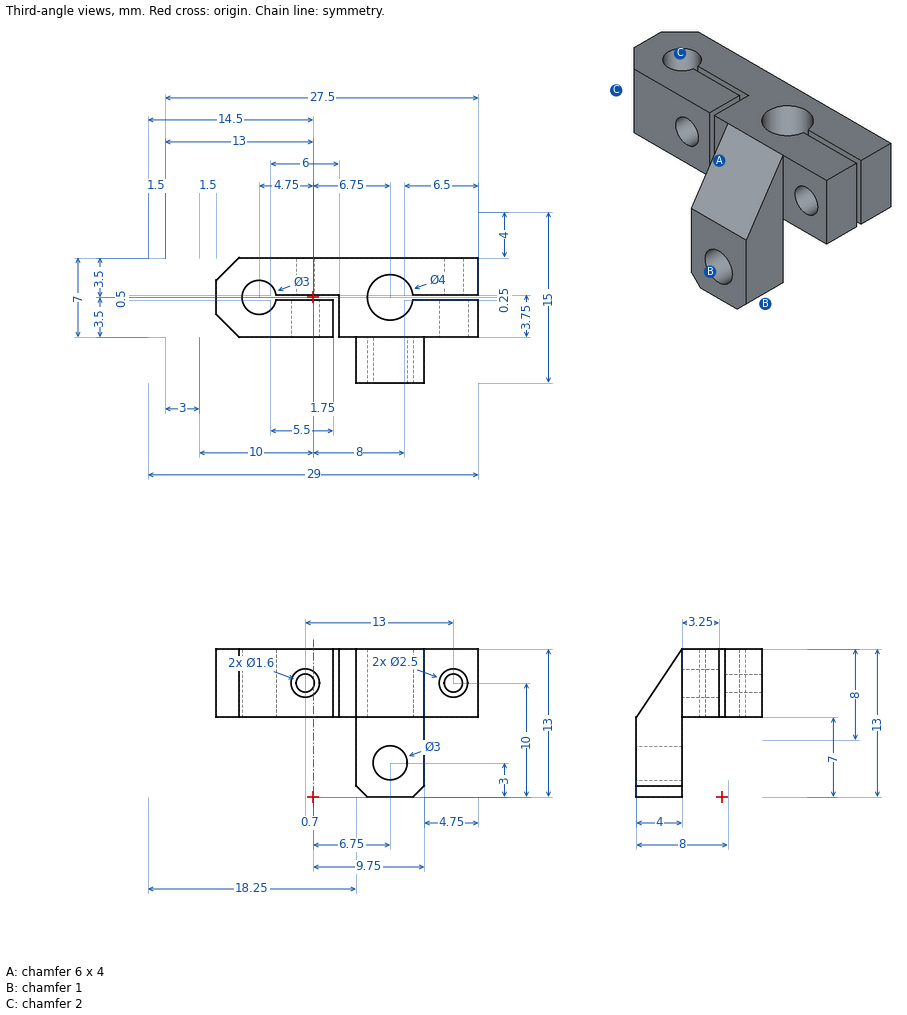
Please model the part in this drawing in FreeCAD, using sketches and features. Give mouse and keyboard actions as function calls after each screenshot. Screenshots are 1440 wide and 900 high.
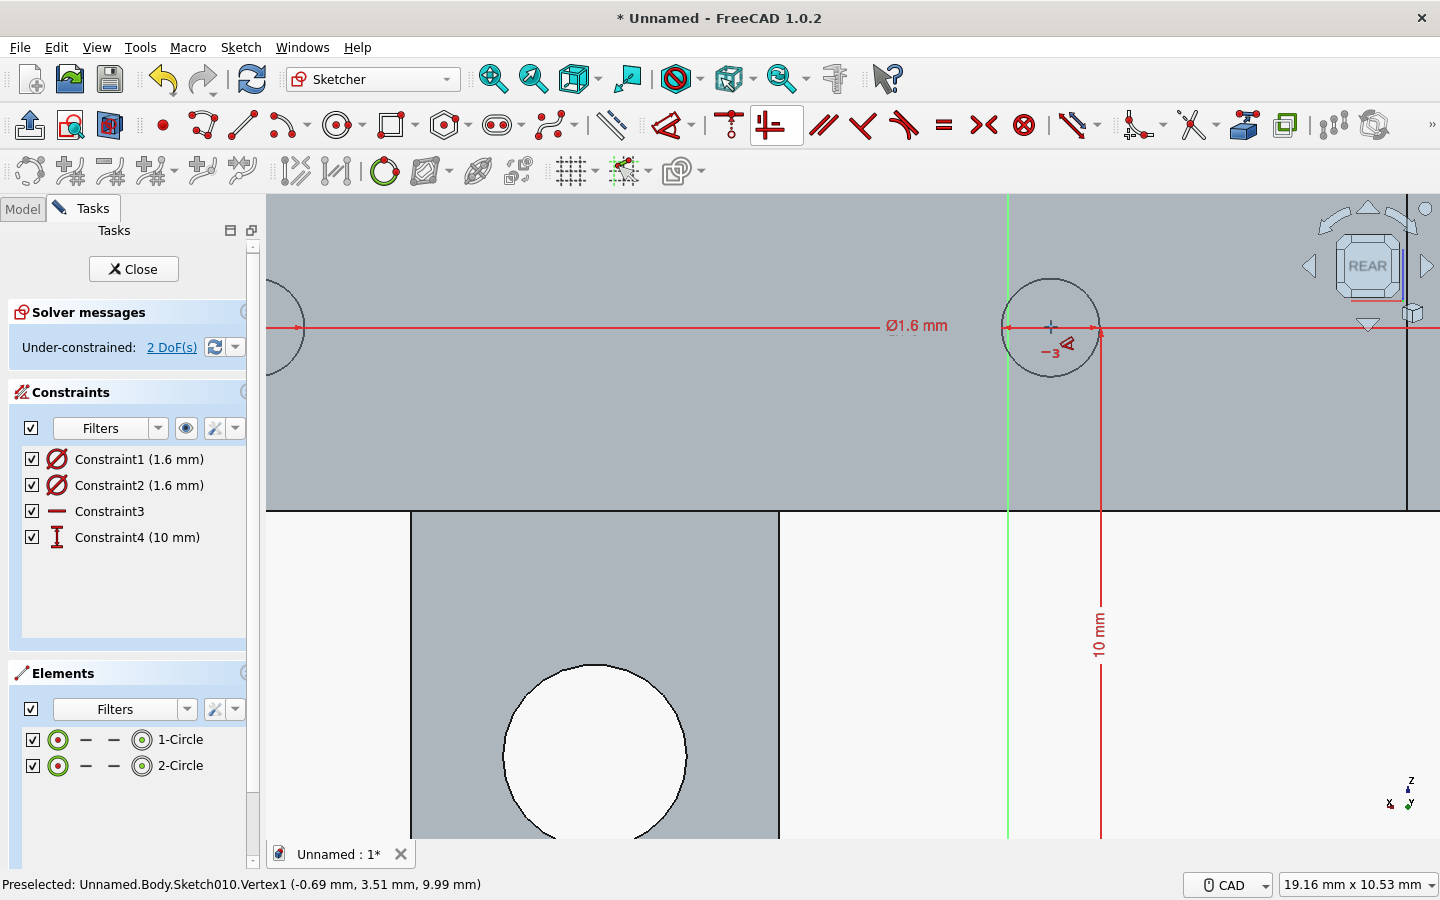
click(1051, 328)
click(1039, 294)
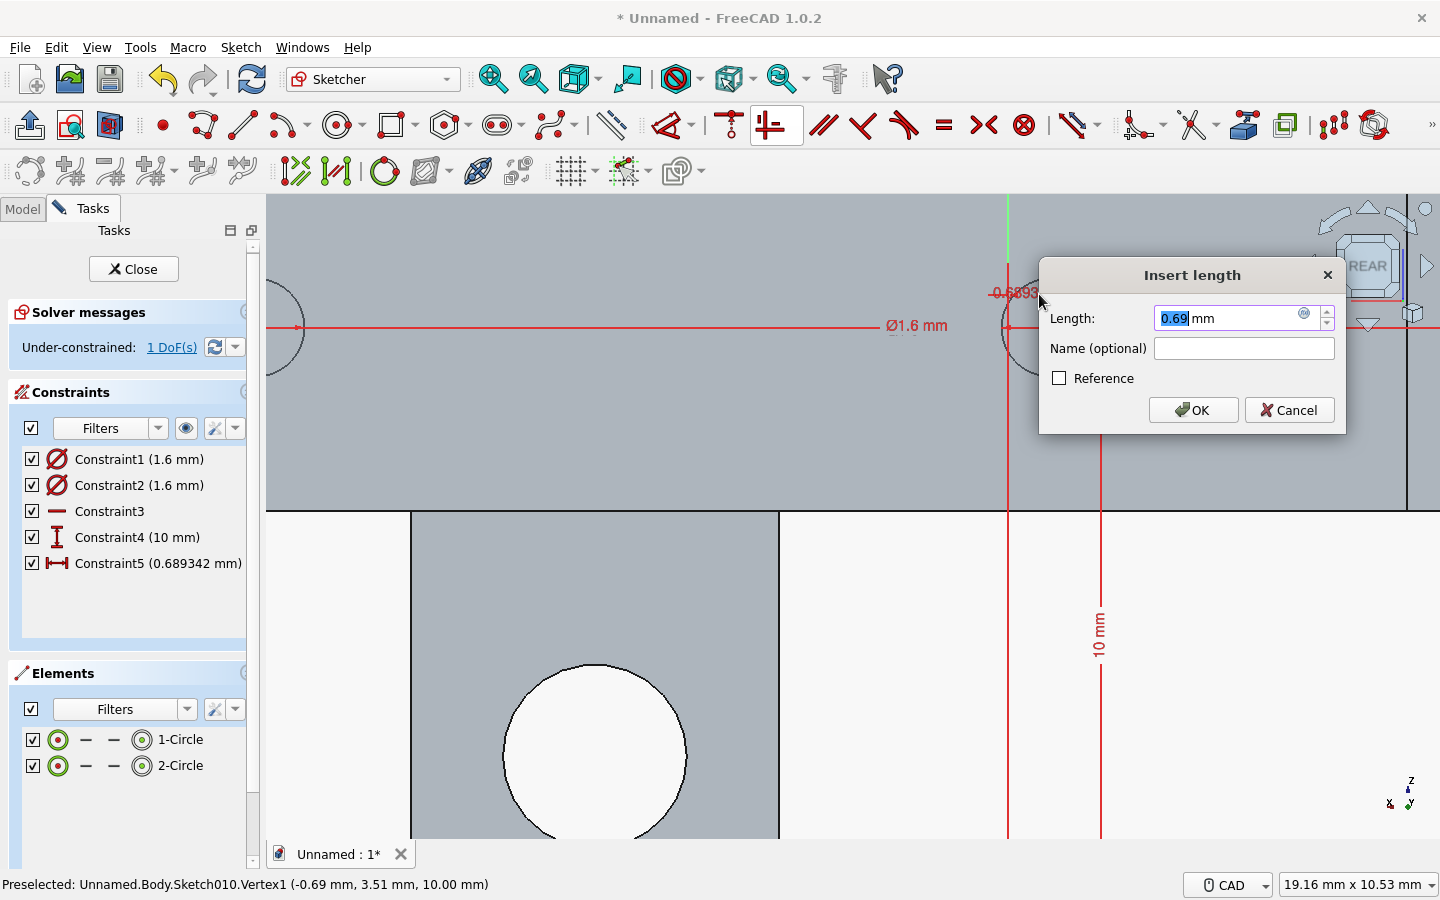
text(0.7)
key(Return)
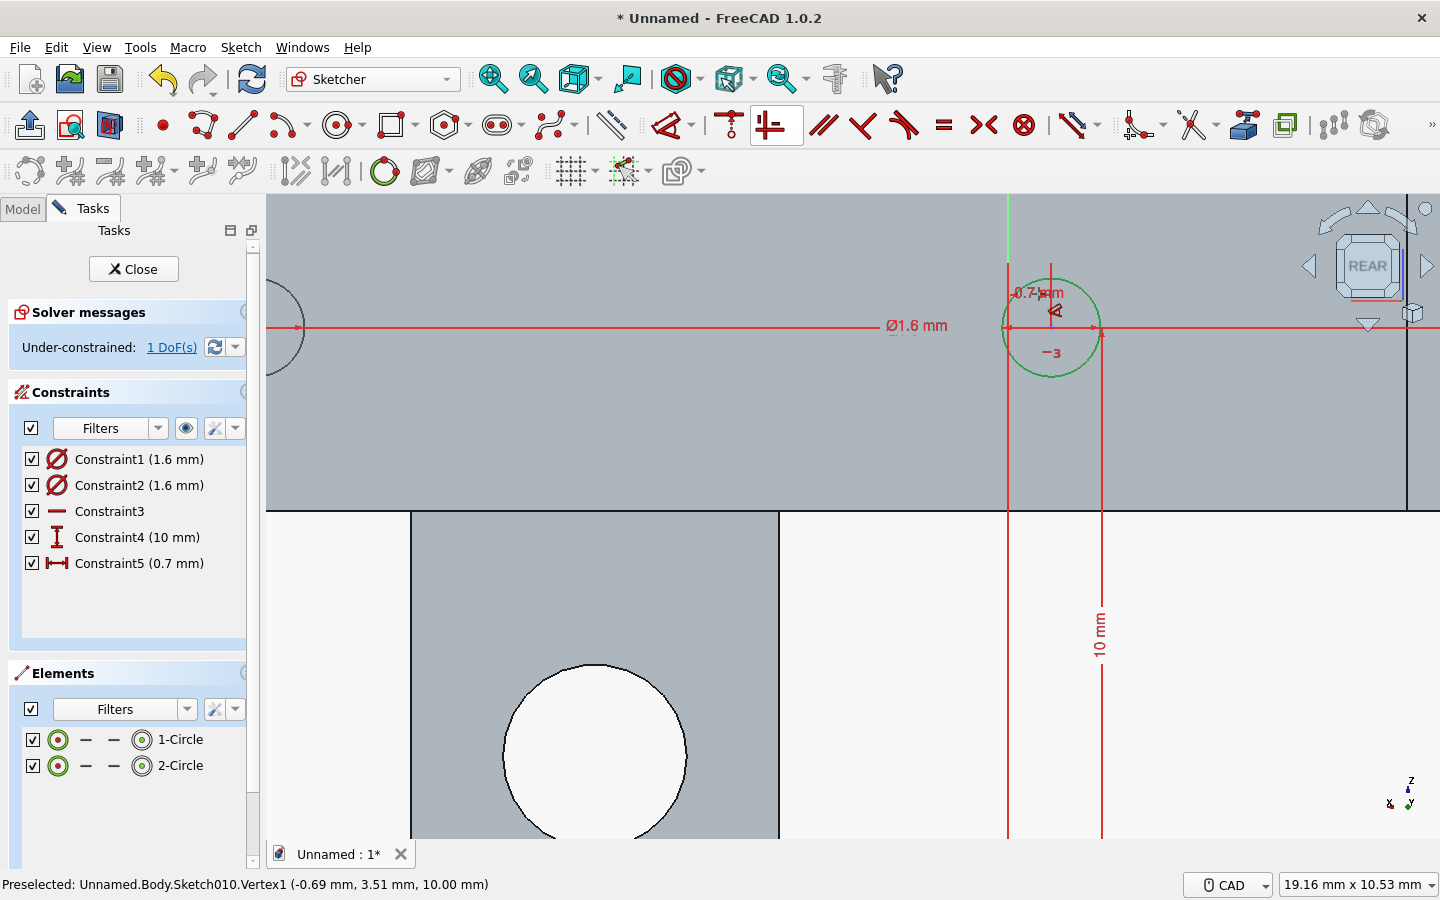
click(1051, 328)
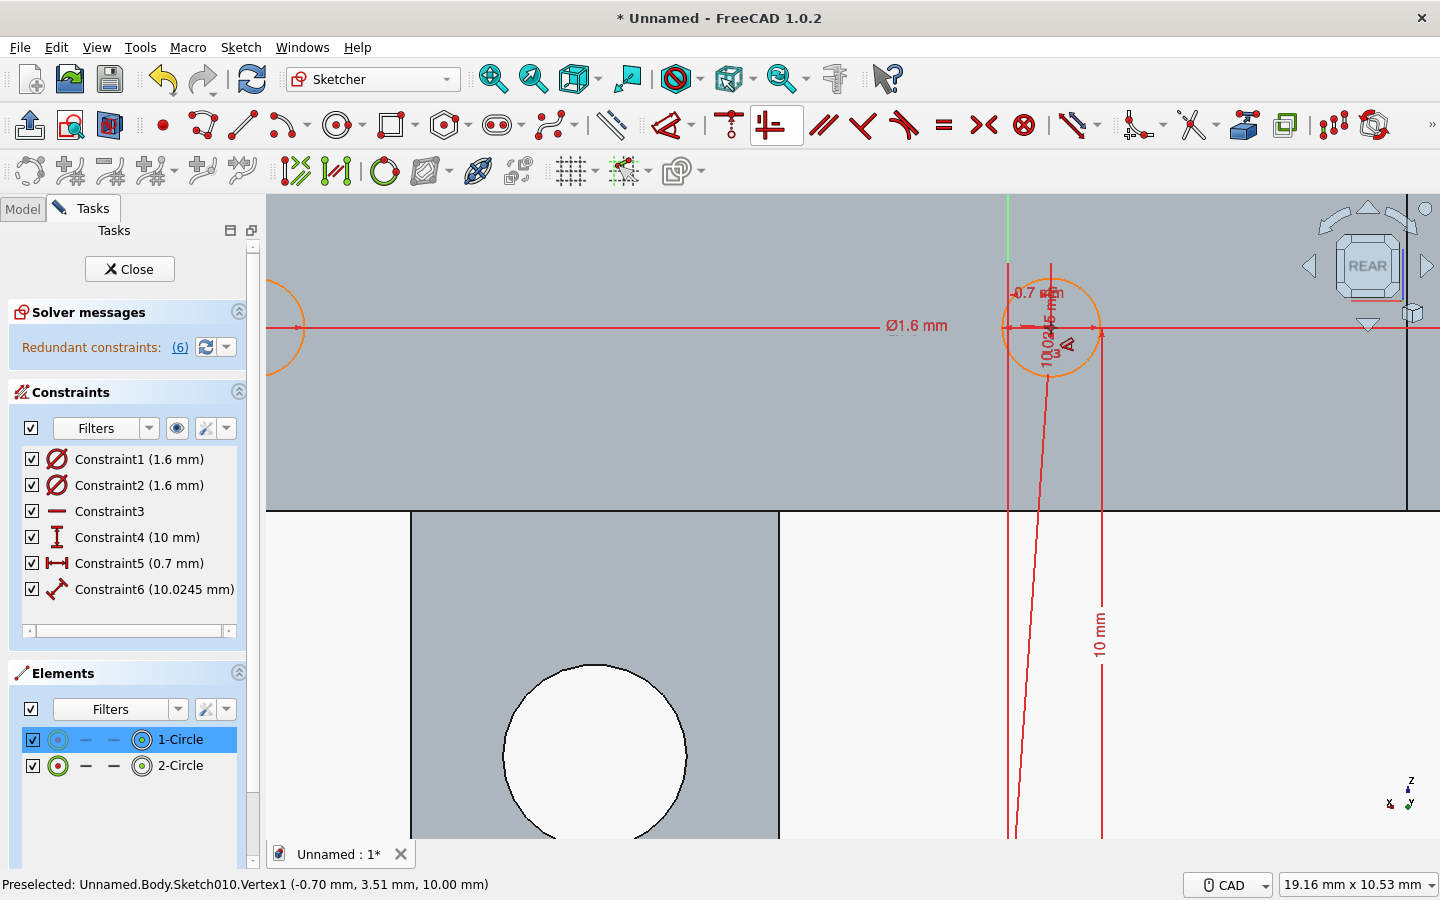
scroll(1052, 328, down, 2)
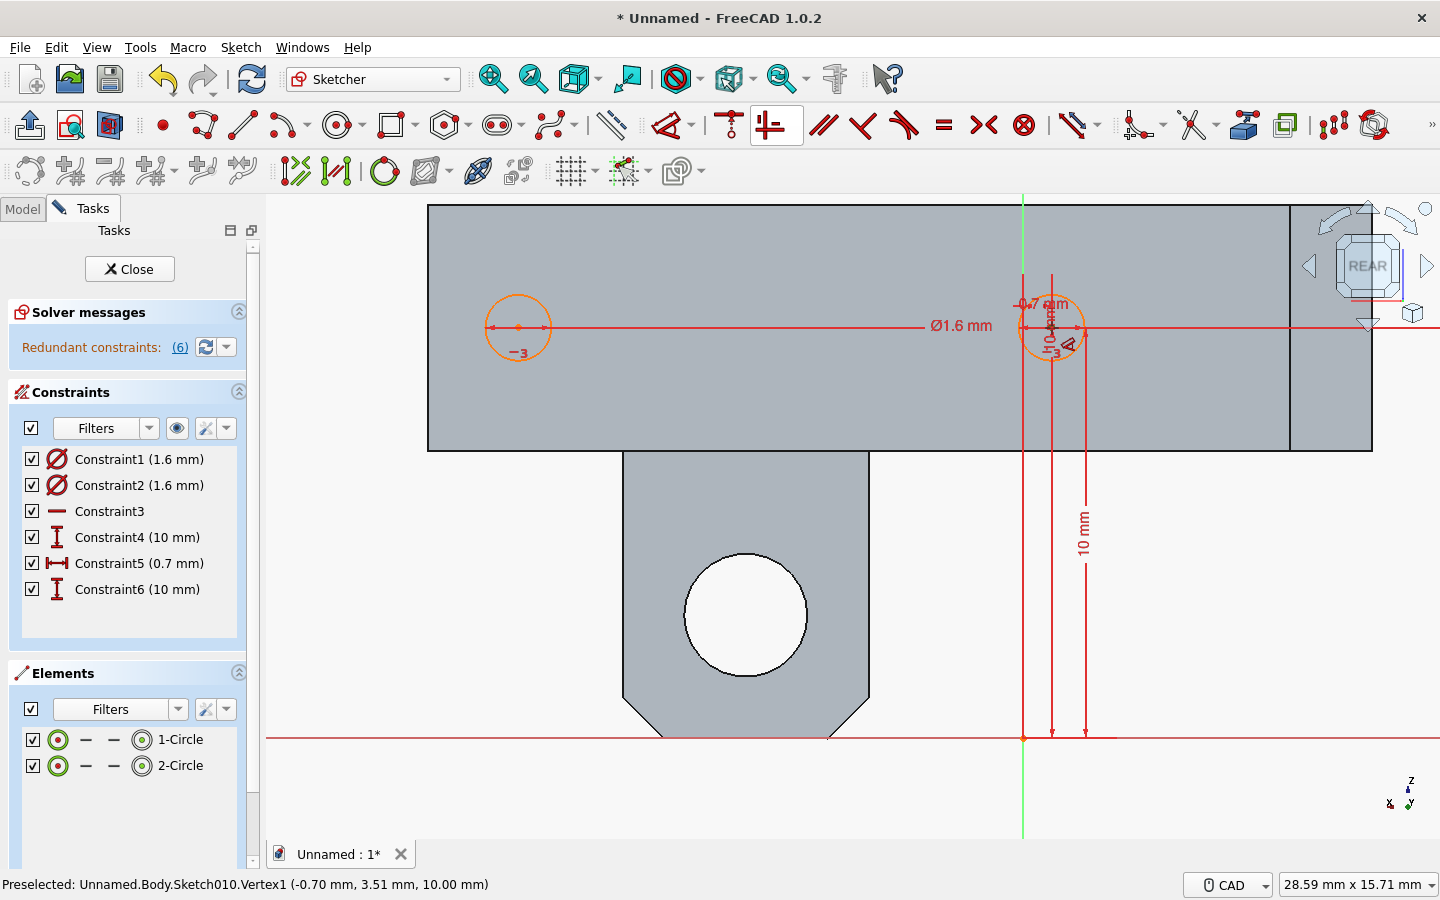
click(518, 328)
click(785, 294)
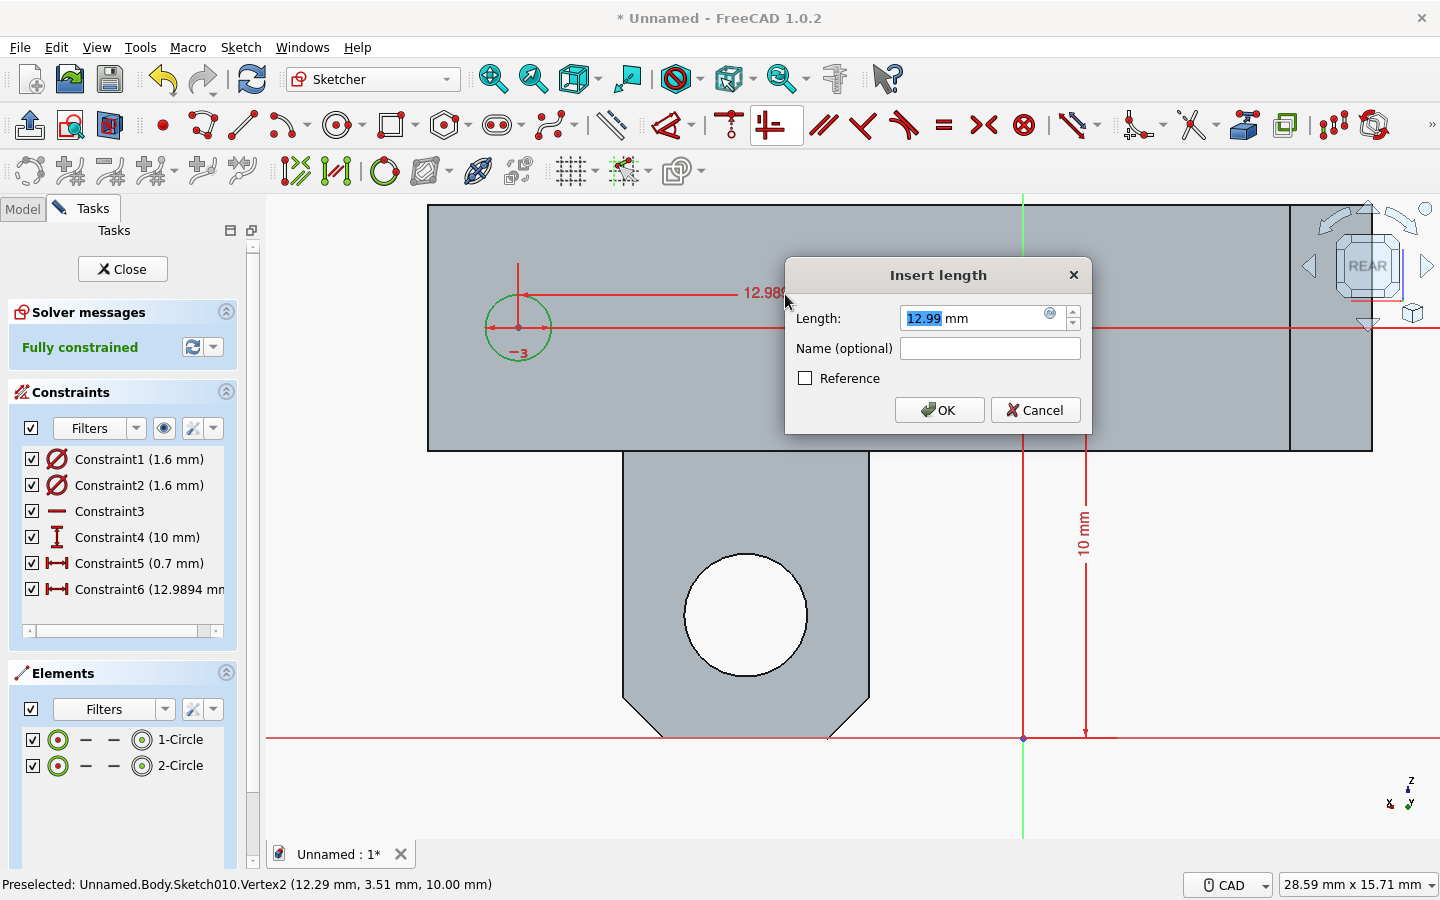
text(13)
key(Return)
key(Escape)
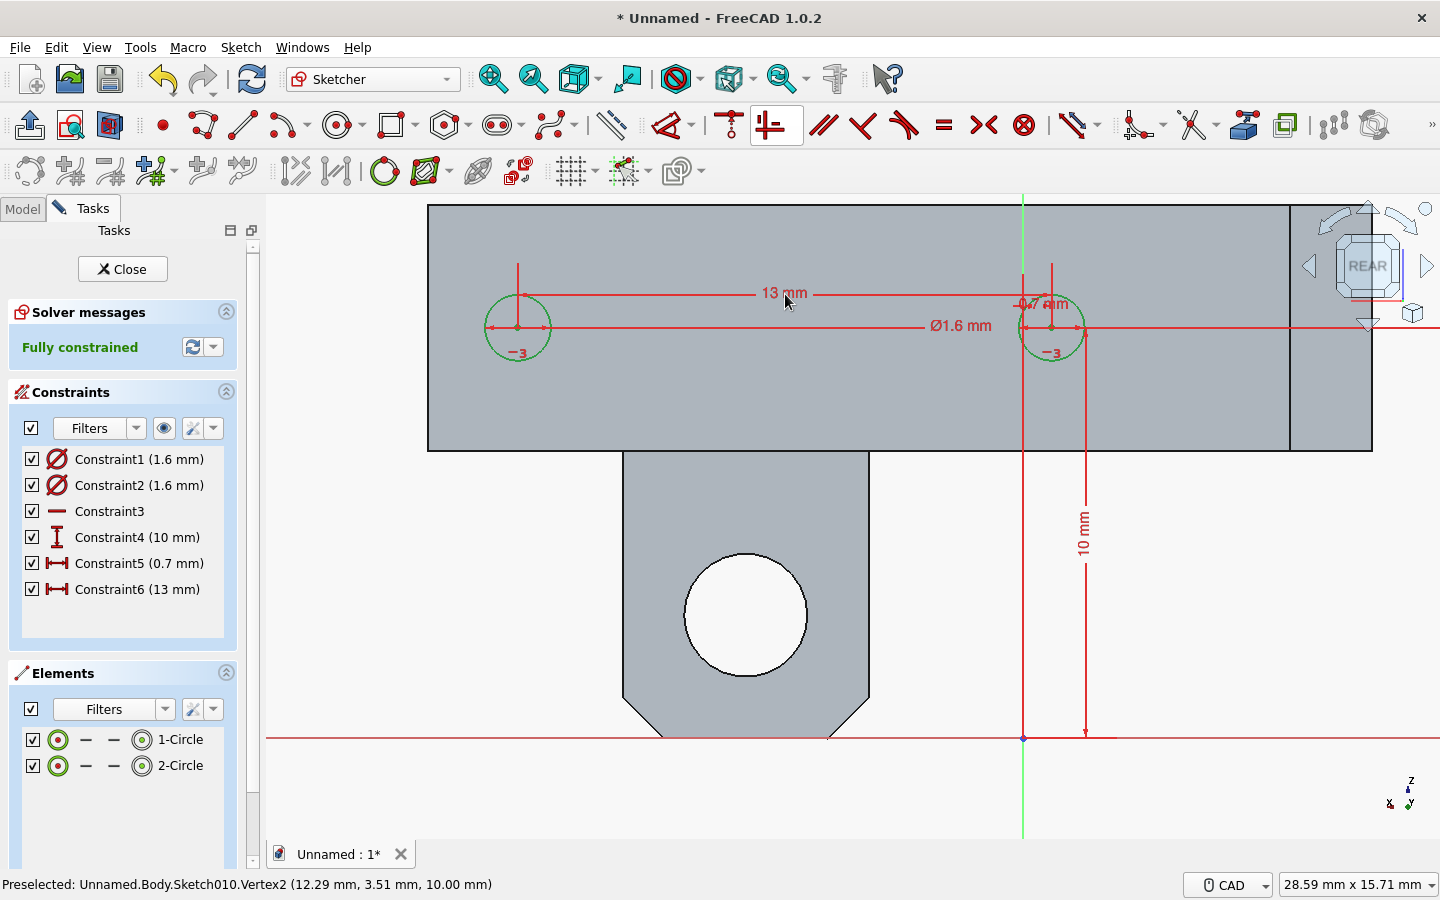
click(123, 269)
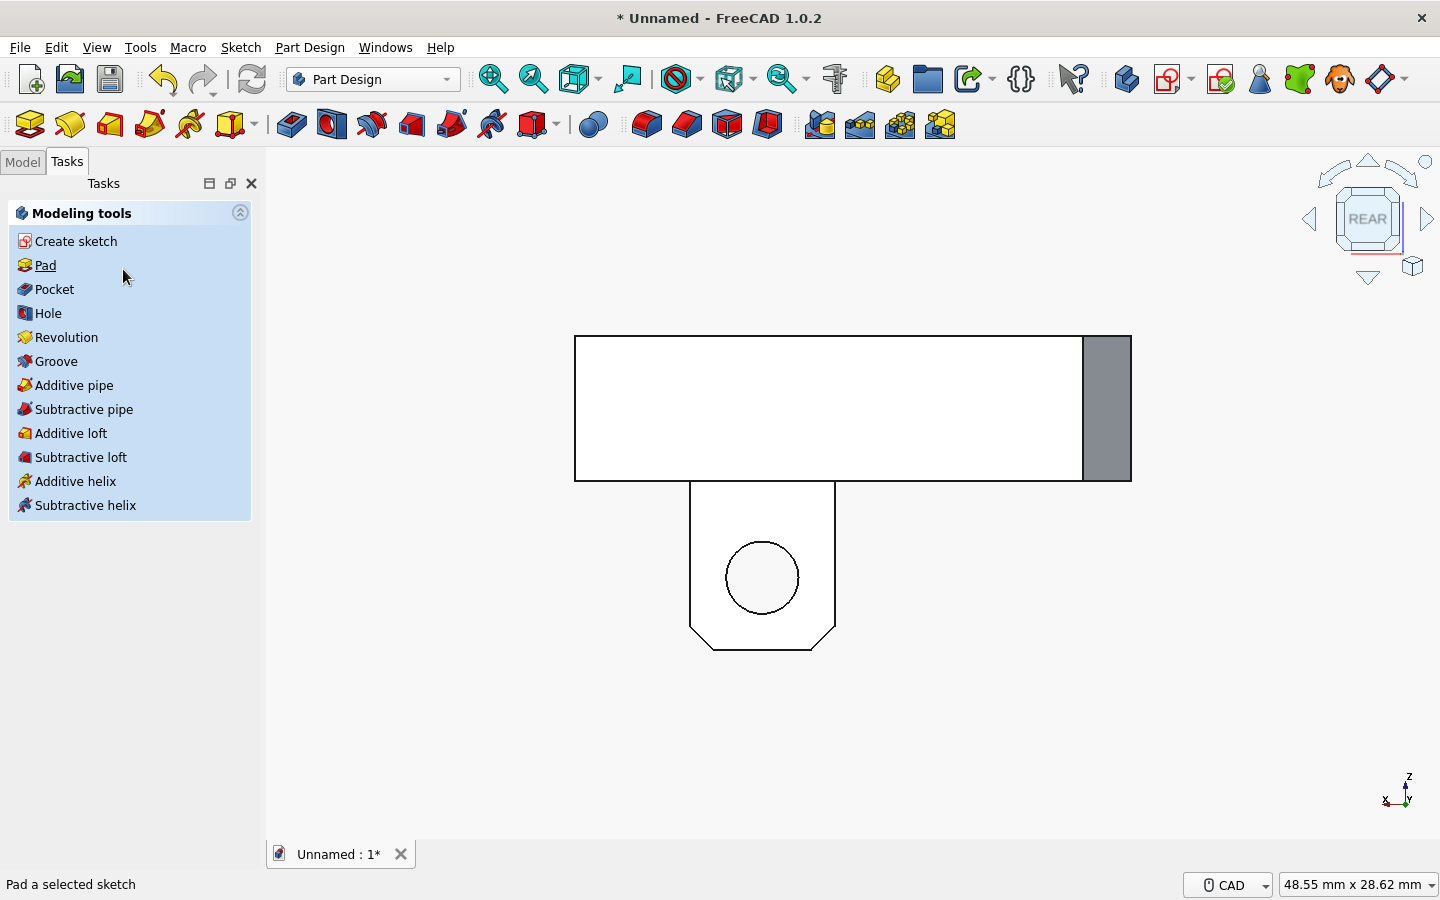
click(292, 124)